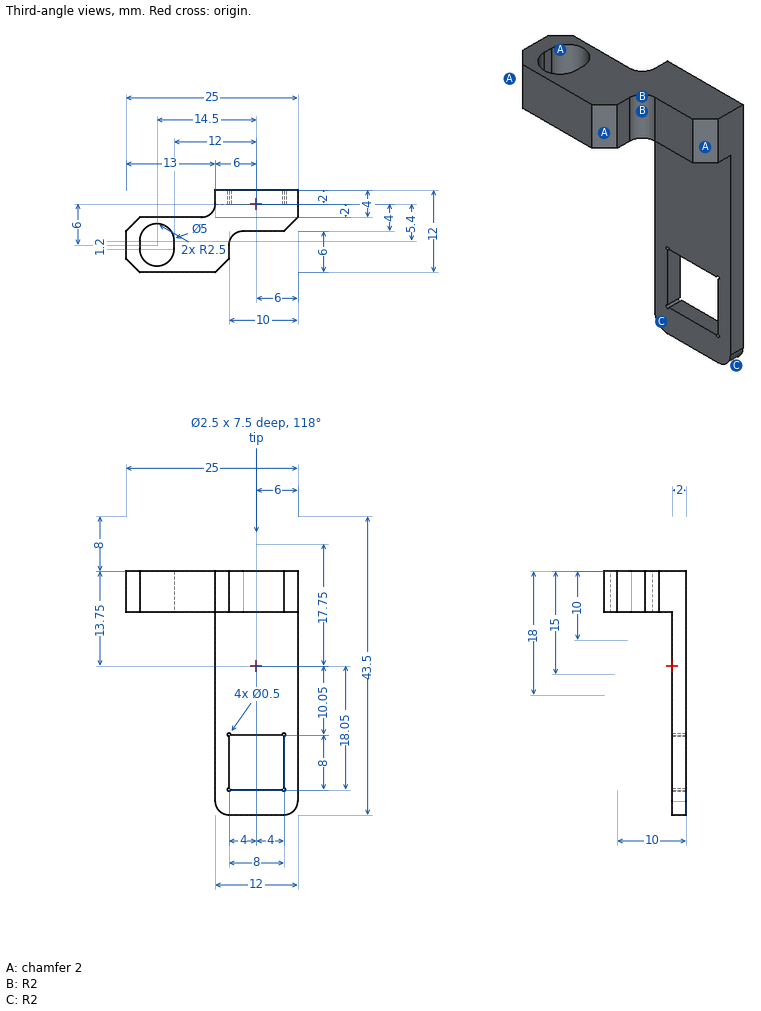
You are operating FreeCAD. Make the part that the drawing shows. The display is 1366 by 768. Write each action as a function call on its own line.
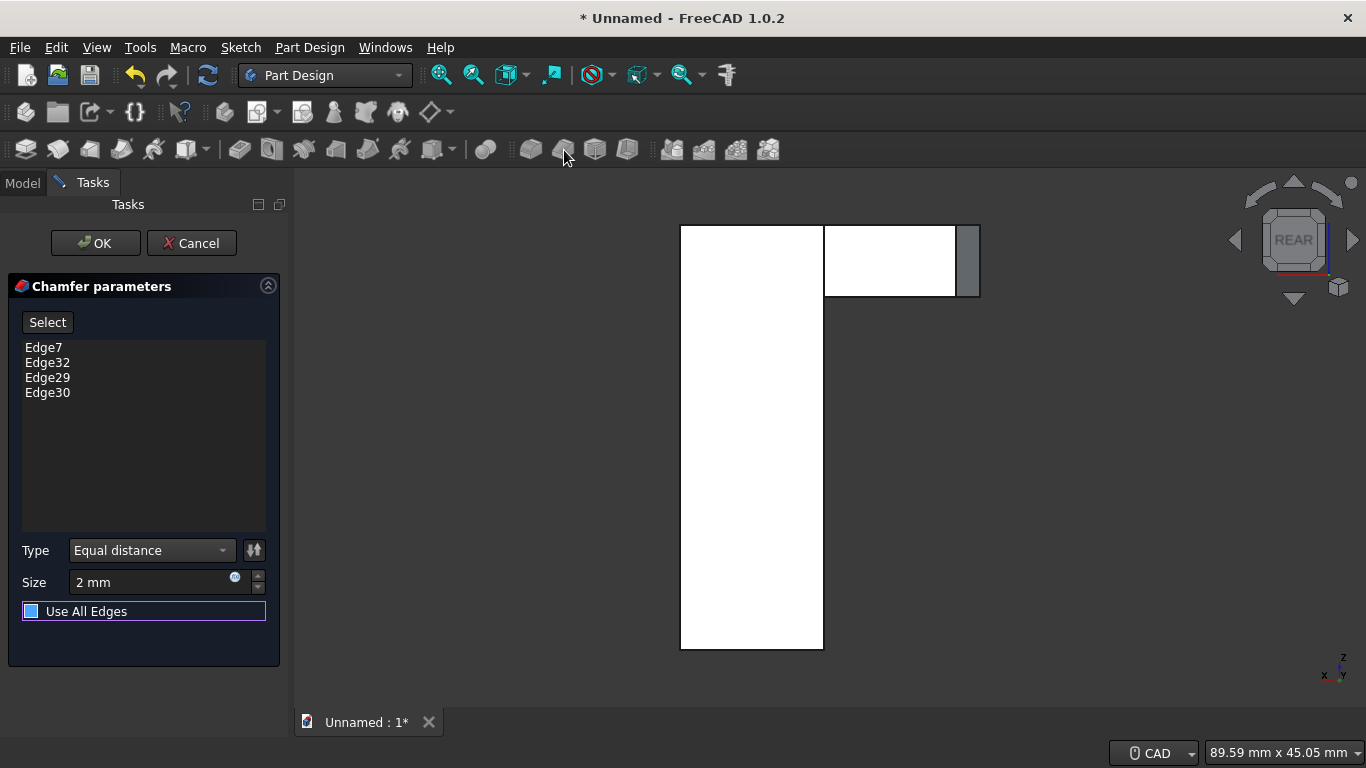
click(96, 243)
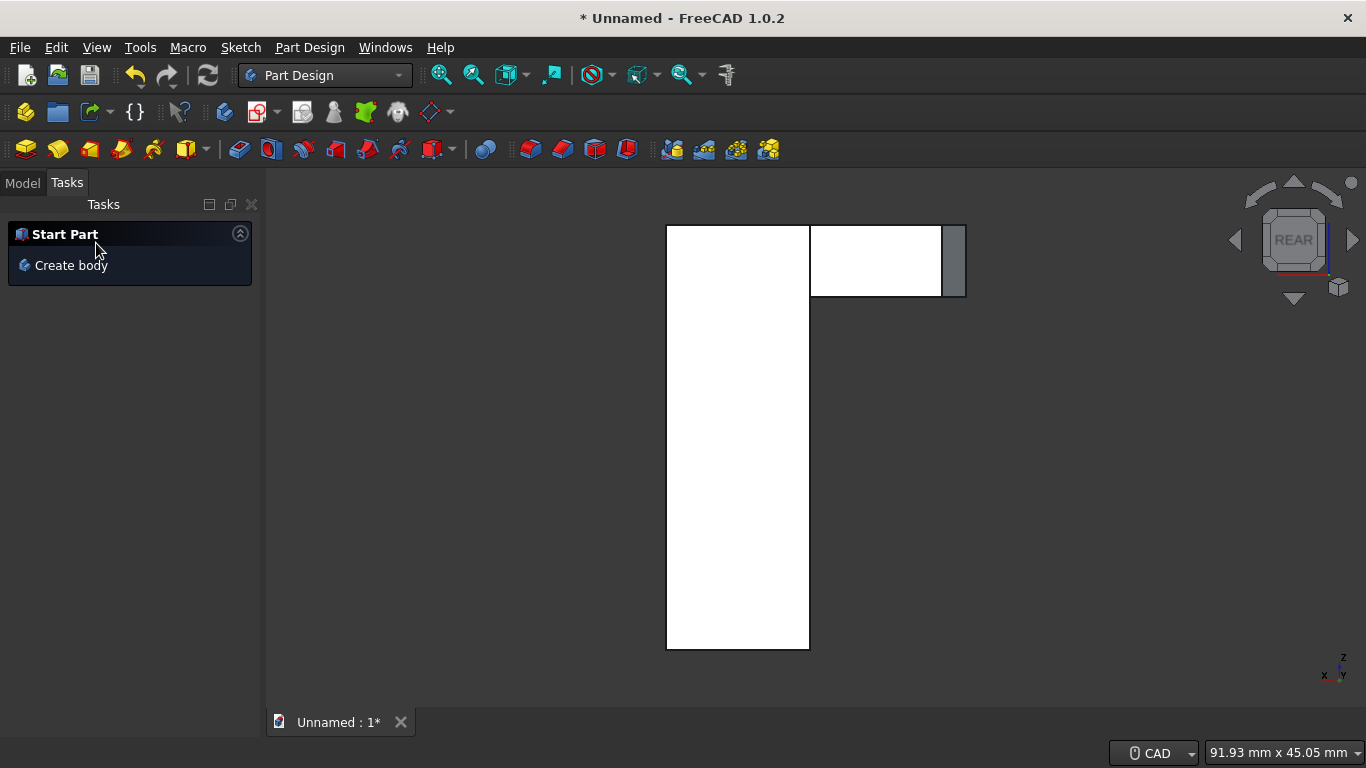
key(0)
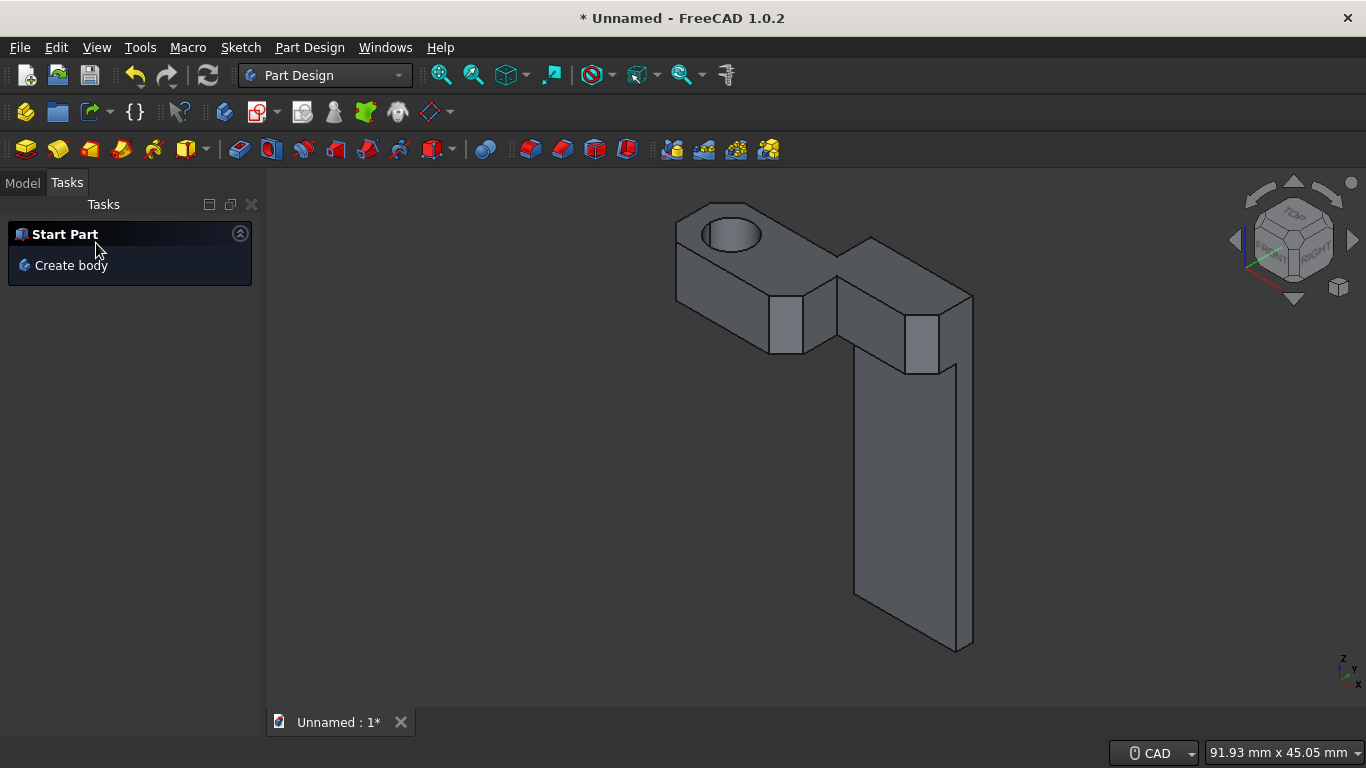
key(2)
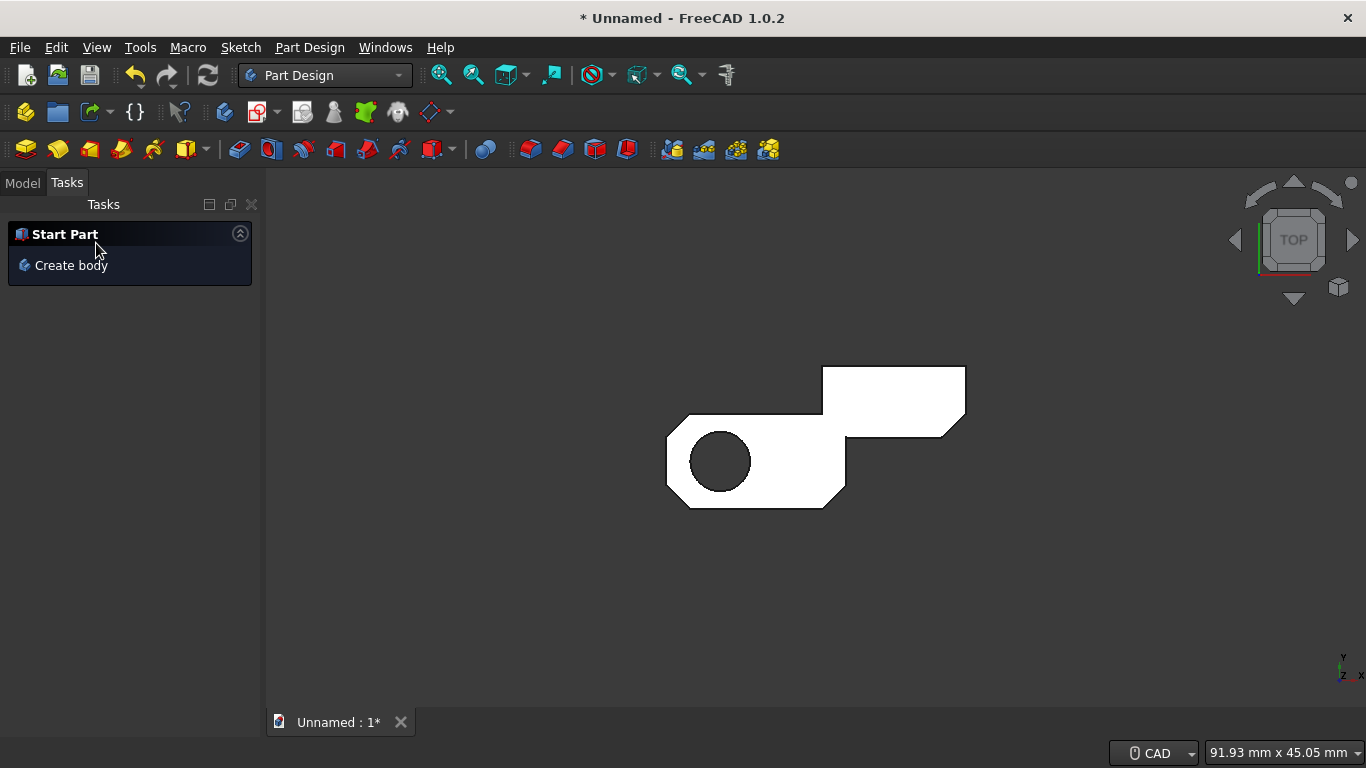
click(442, 76)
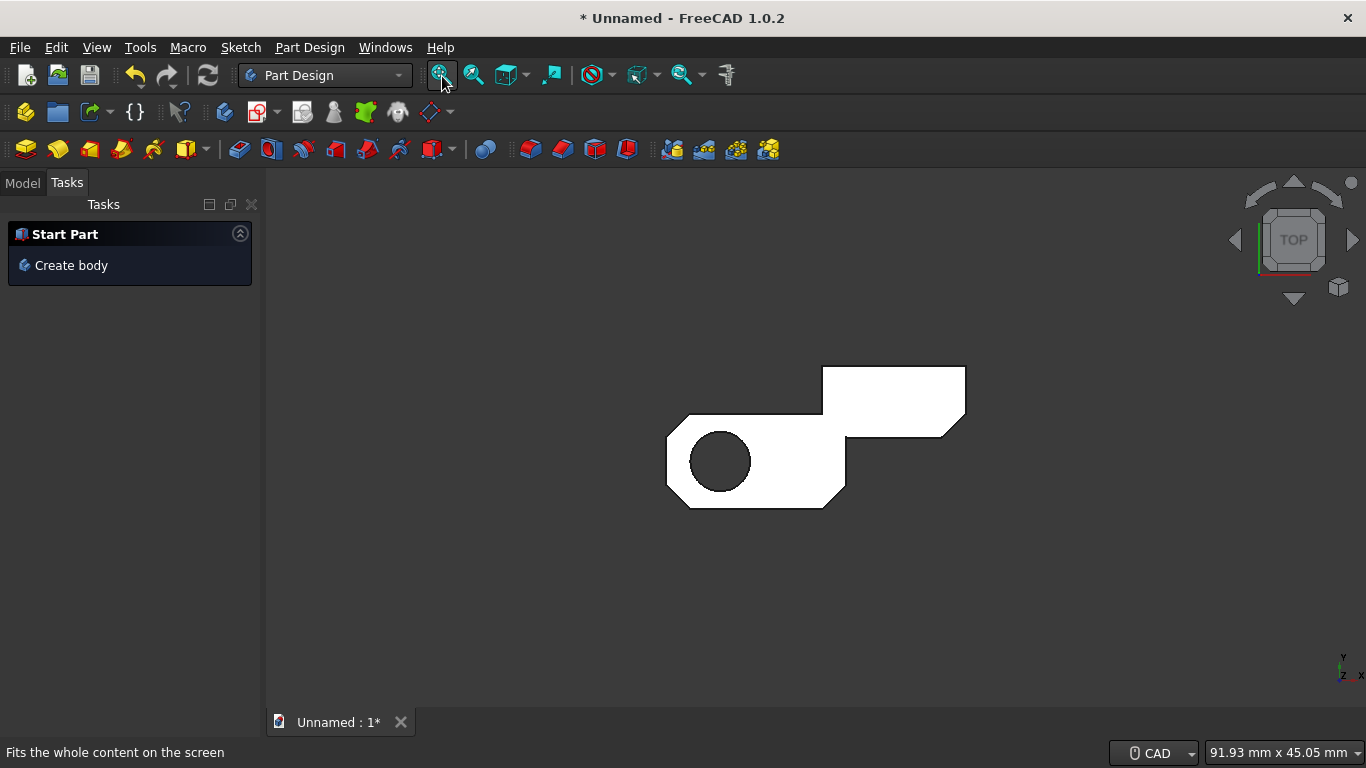
key(1)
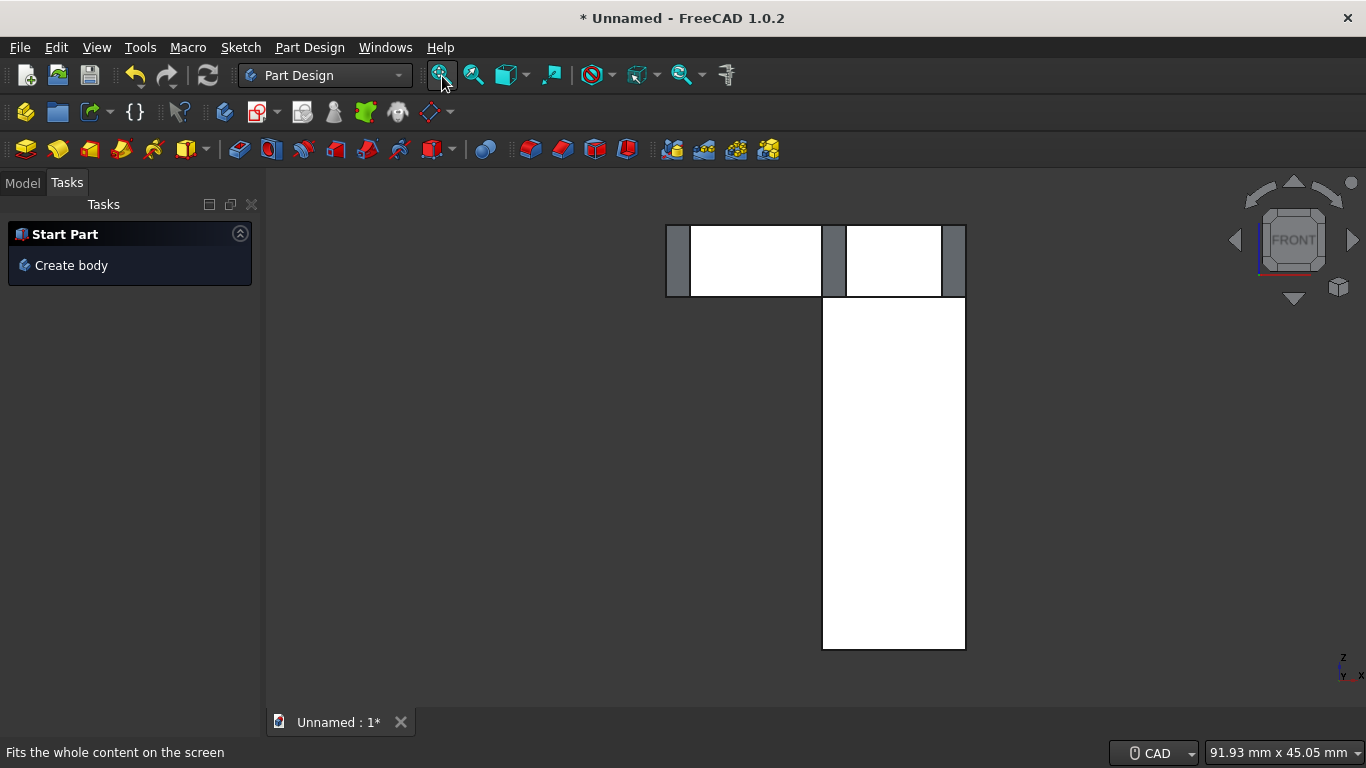
key(3)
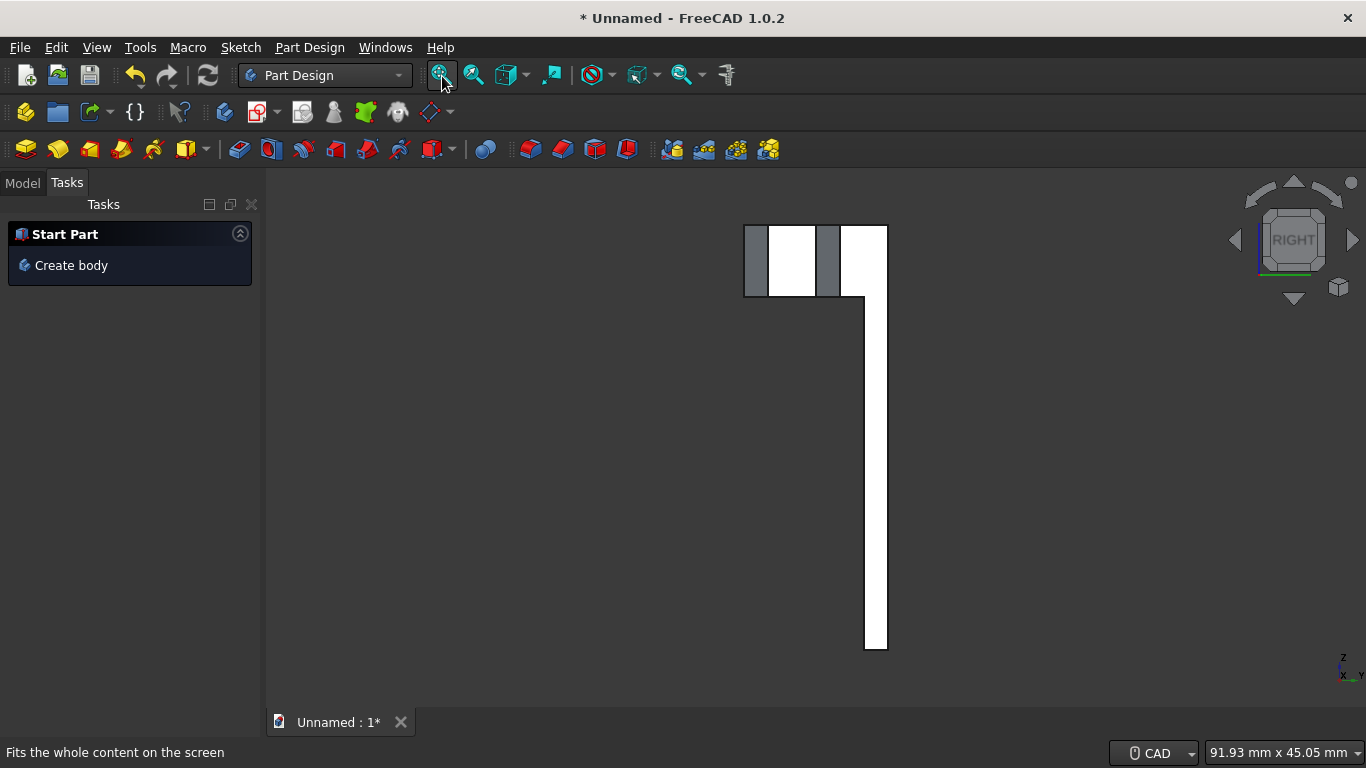
key(5)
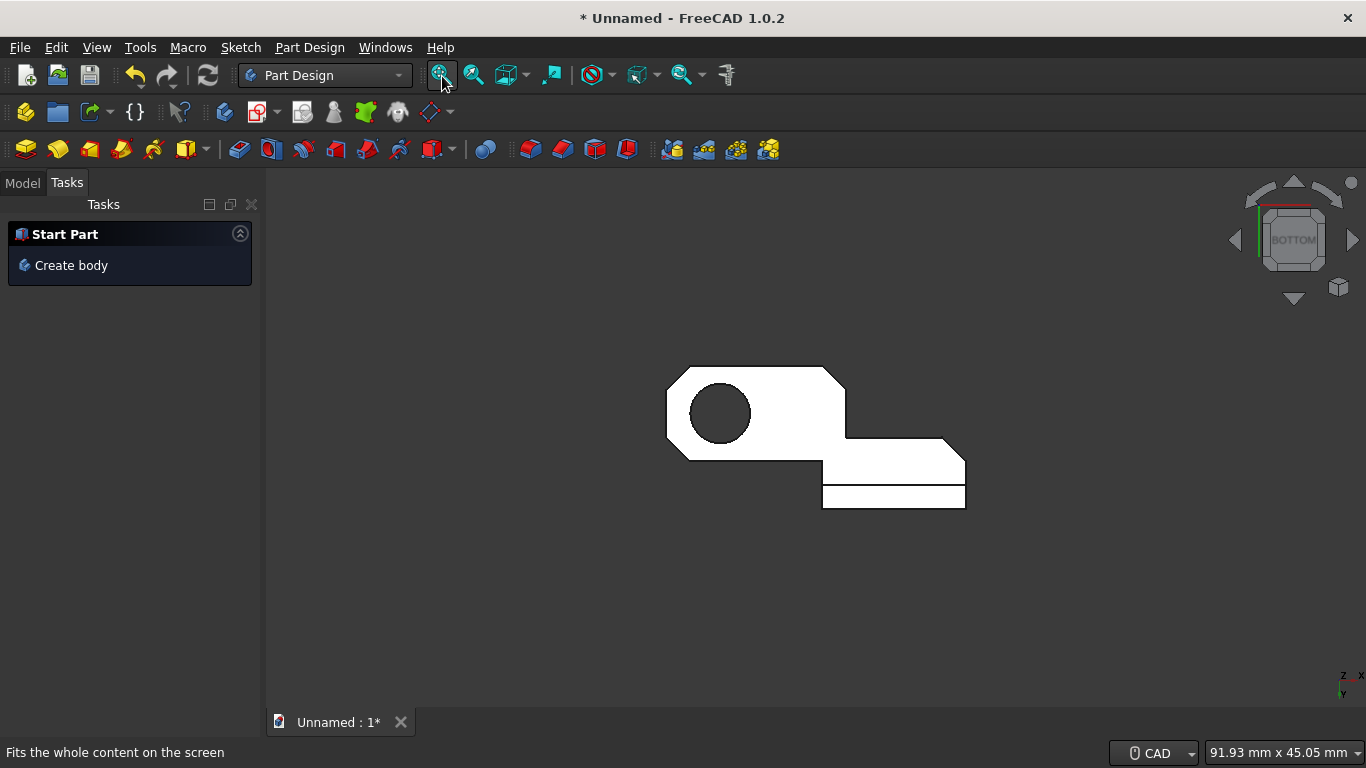
click(442, 76)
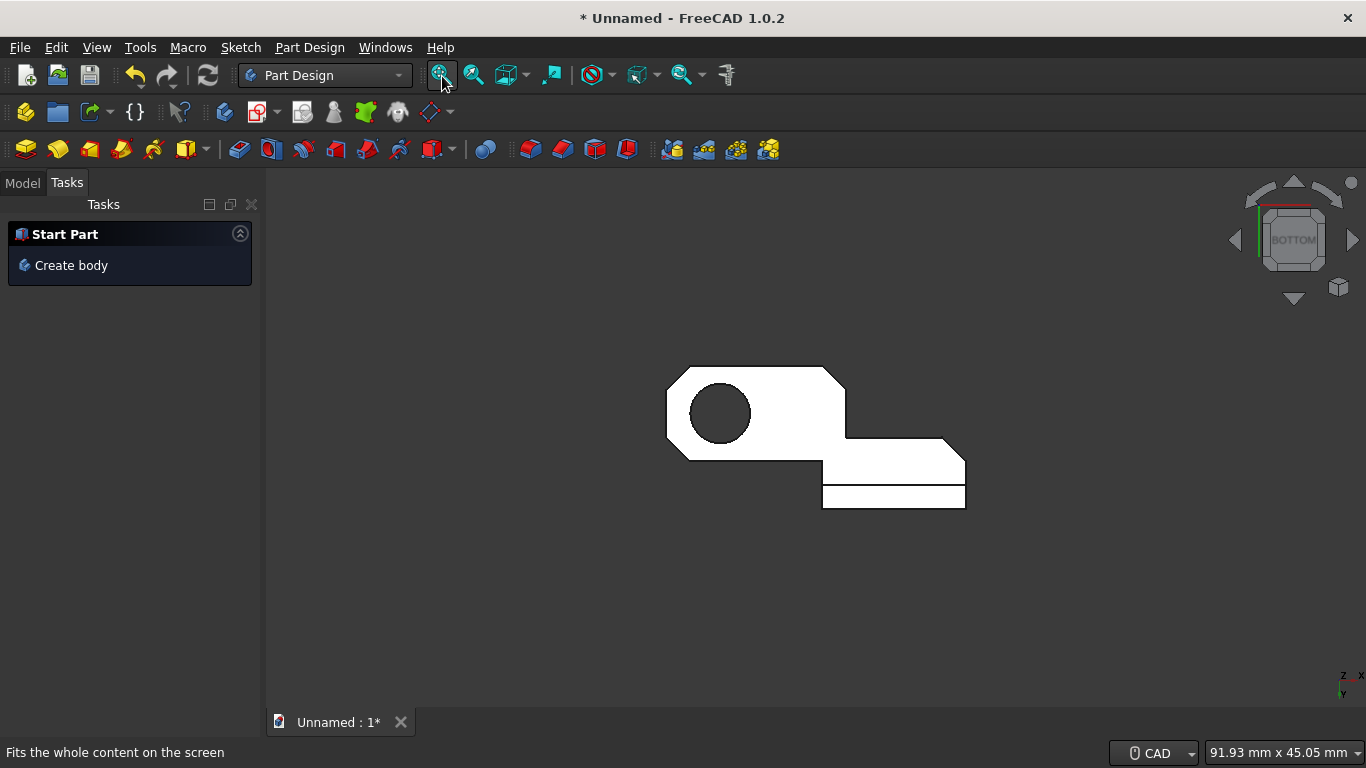
key(4)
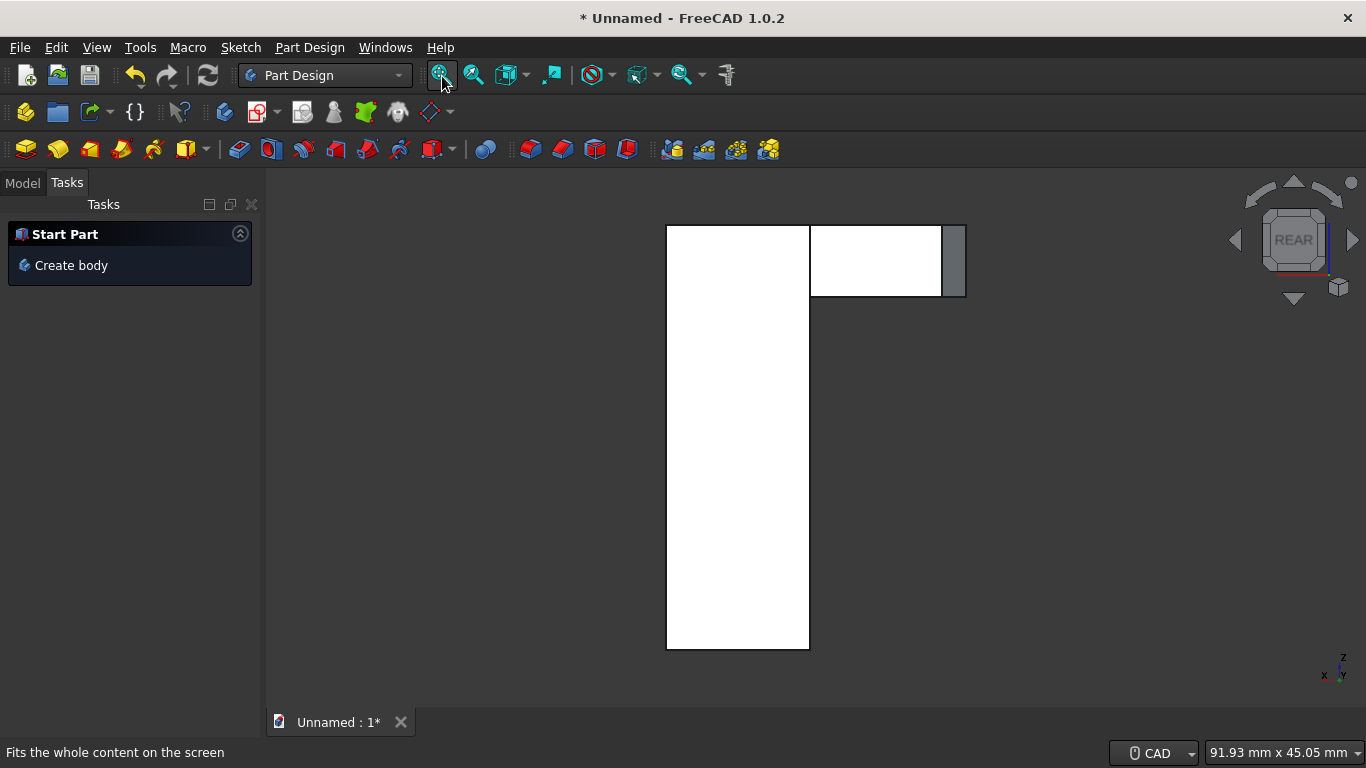
key(6)